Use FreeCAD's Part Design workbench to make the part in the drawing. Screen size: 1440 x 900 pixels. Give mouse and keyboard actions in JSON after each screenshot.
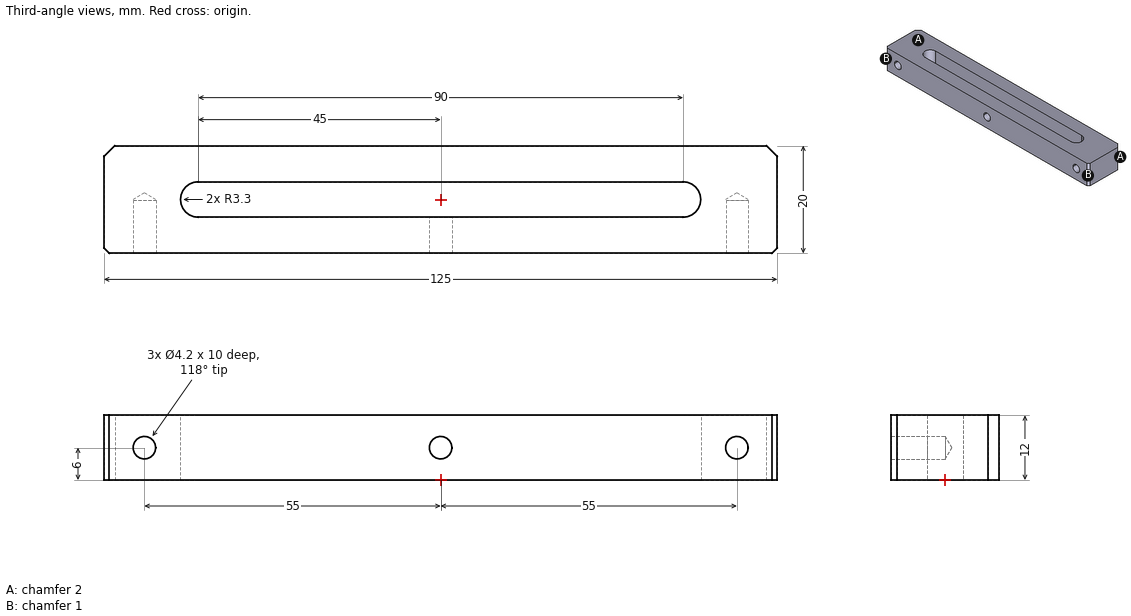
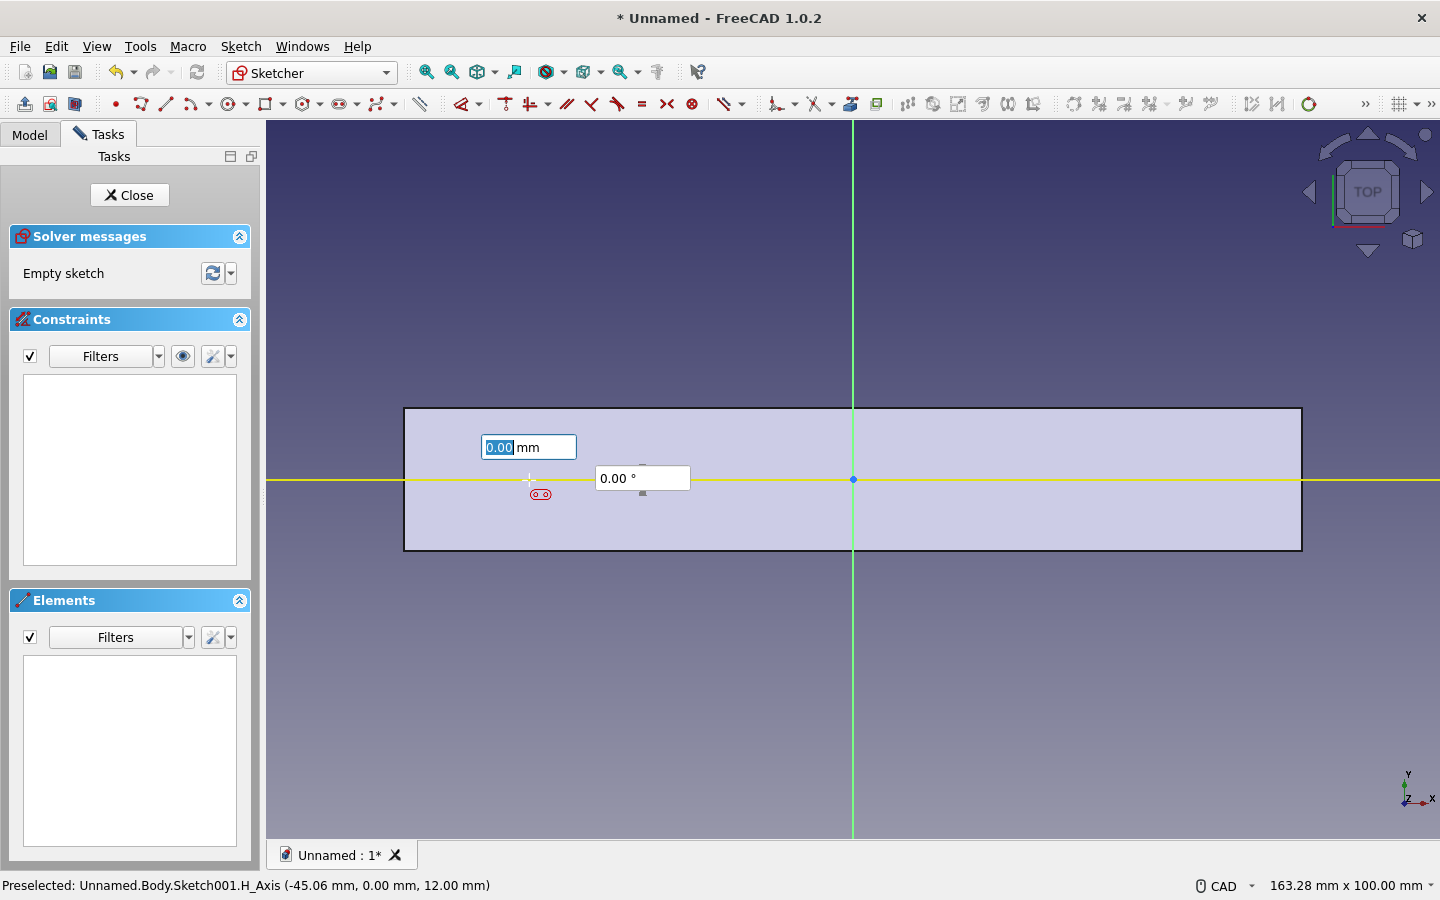
{"action": "left_click", "coordinate": [1177, 470]}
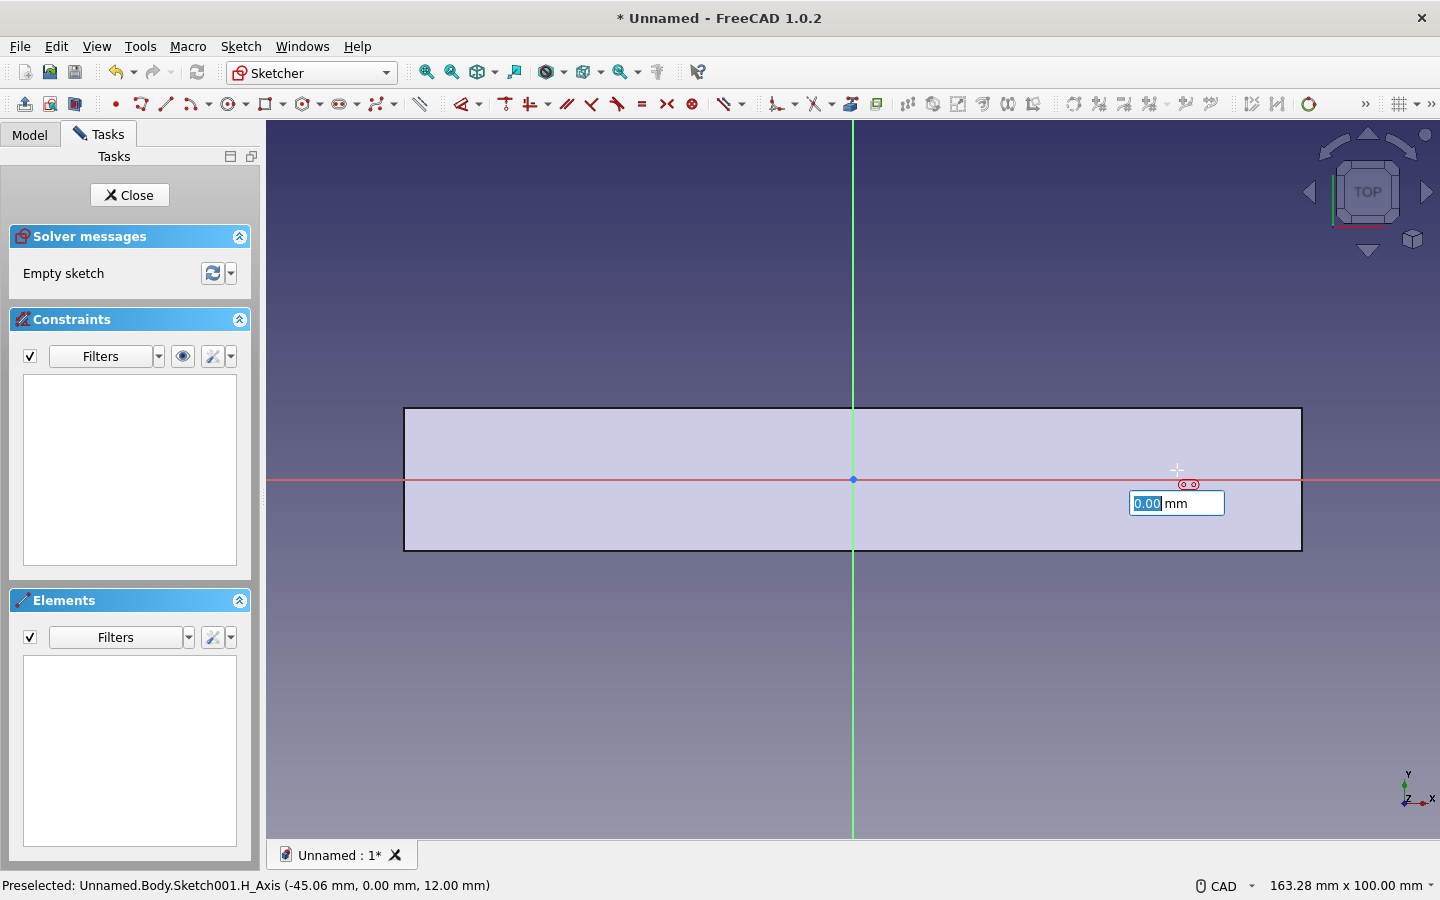
{"action": "left_click", "coordinate": [950, 456]}
{"action": "key", "text": "Escape"}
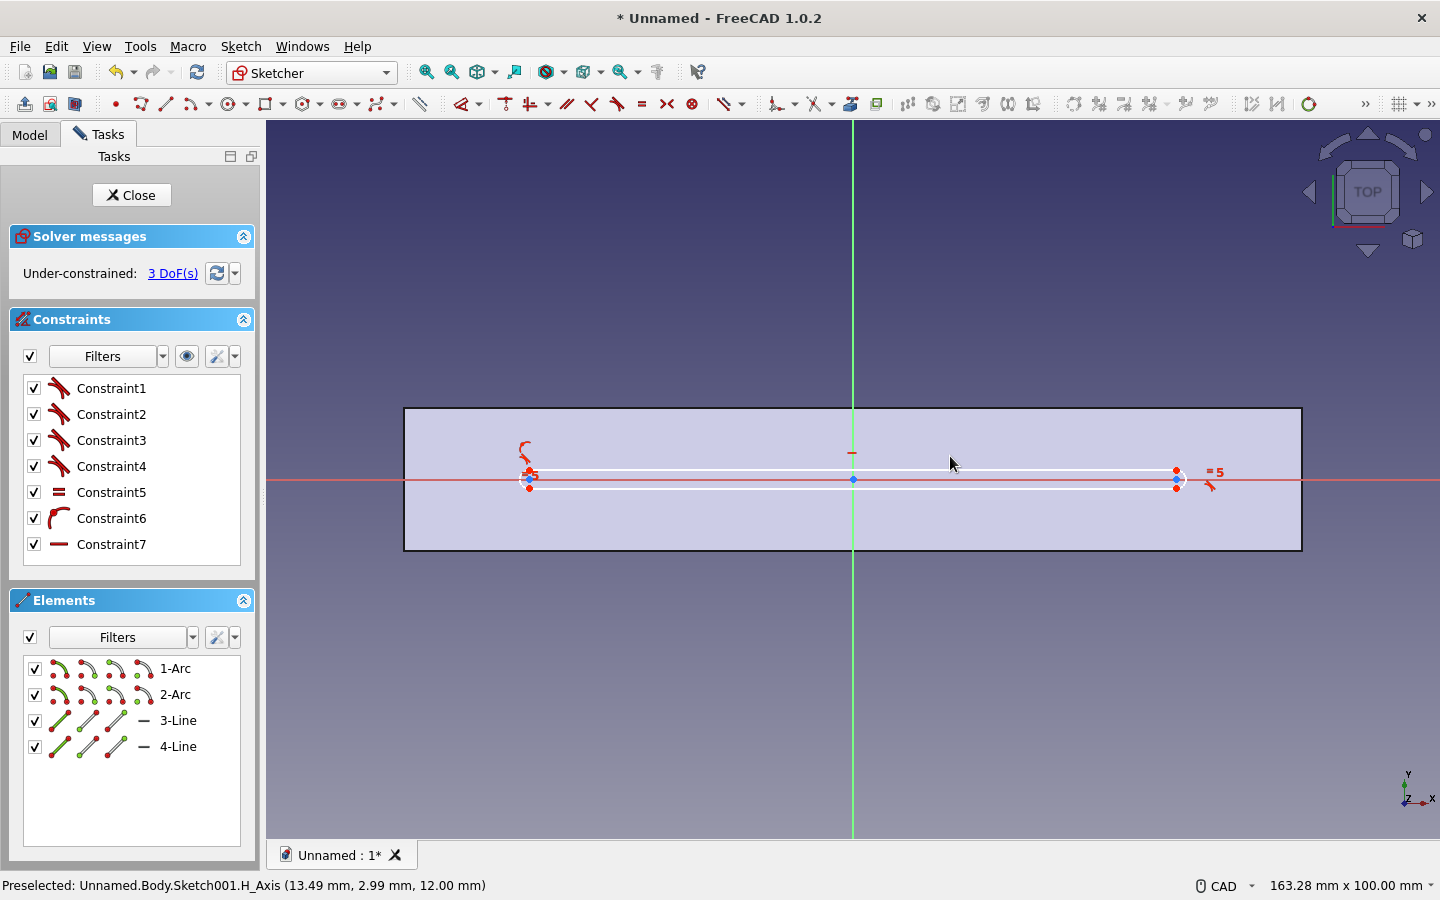
{"action": "key", "text": "d"}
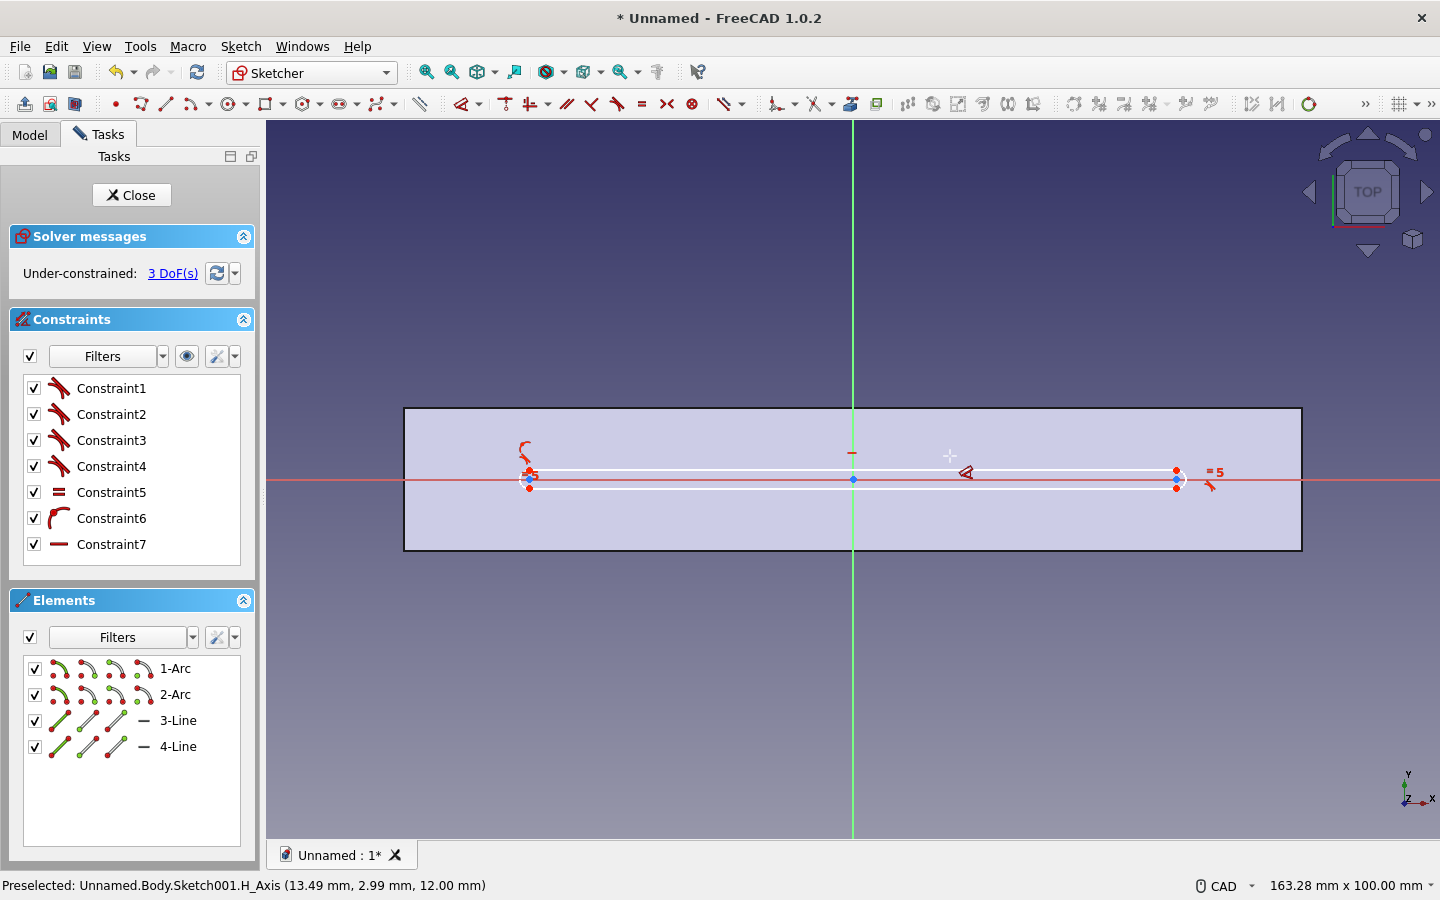
{"action": "scroll", "coordinate": [520, 479], "scroll_direction": "up", "scroll_amount": 3}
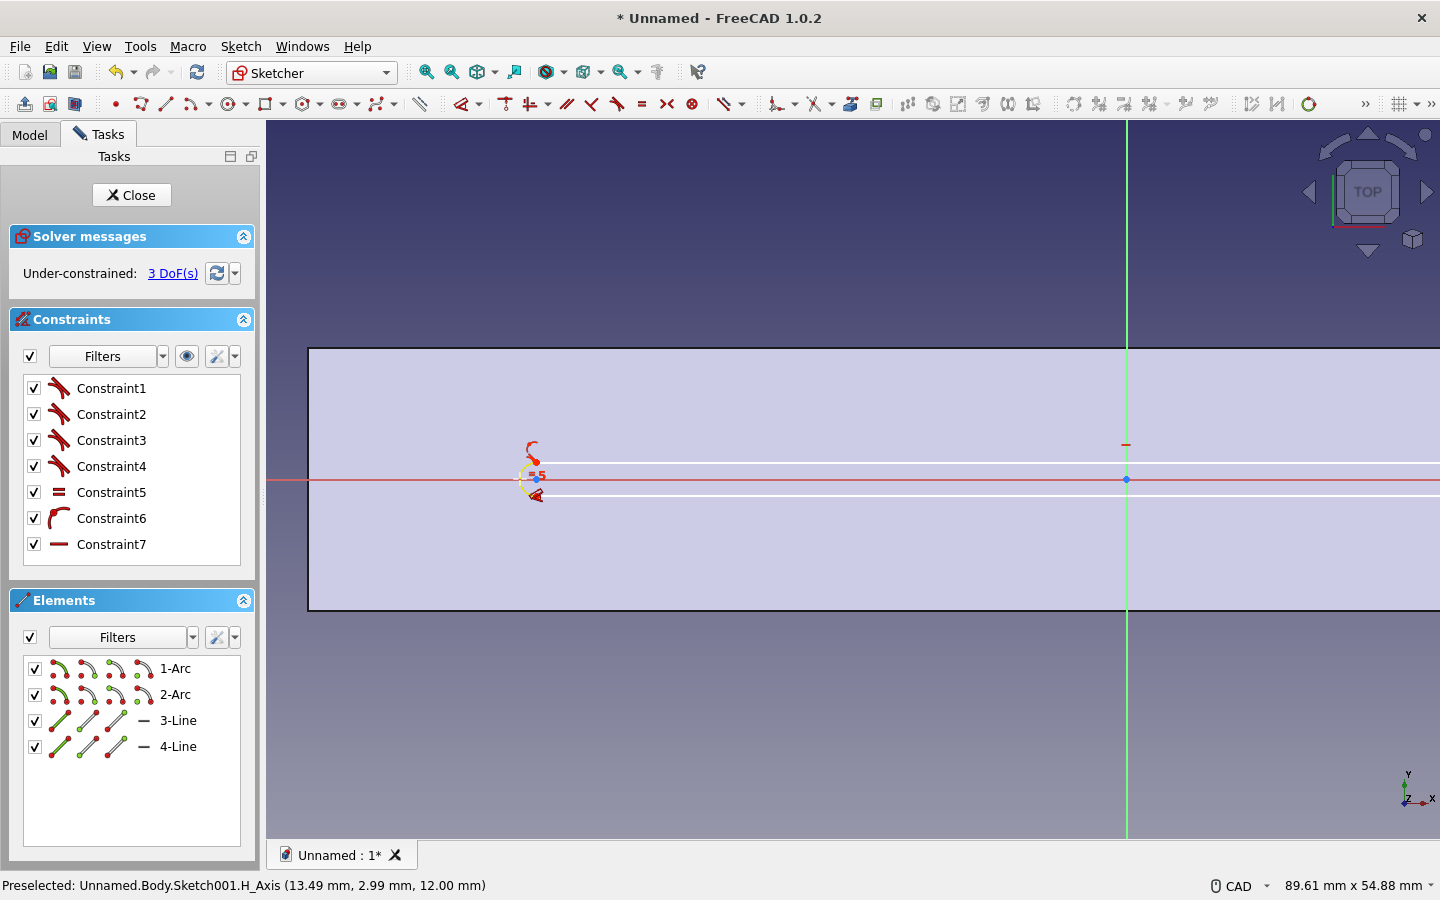
{"action": "left_click", "coordinate": [520, 479]}
{"action": "left_click", "coordinate": [495, 455]}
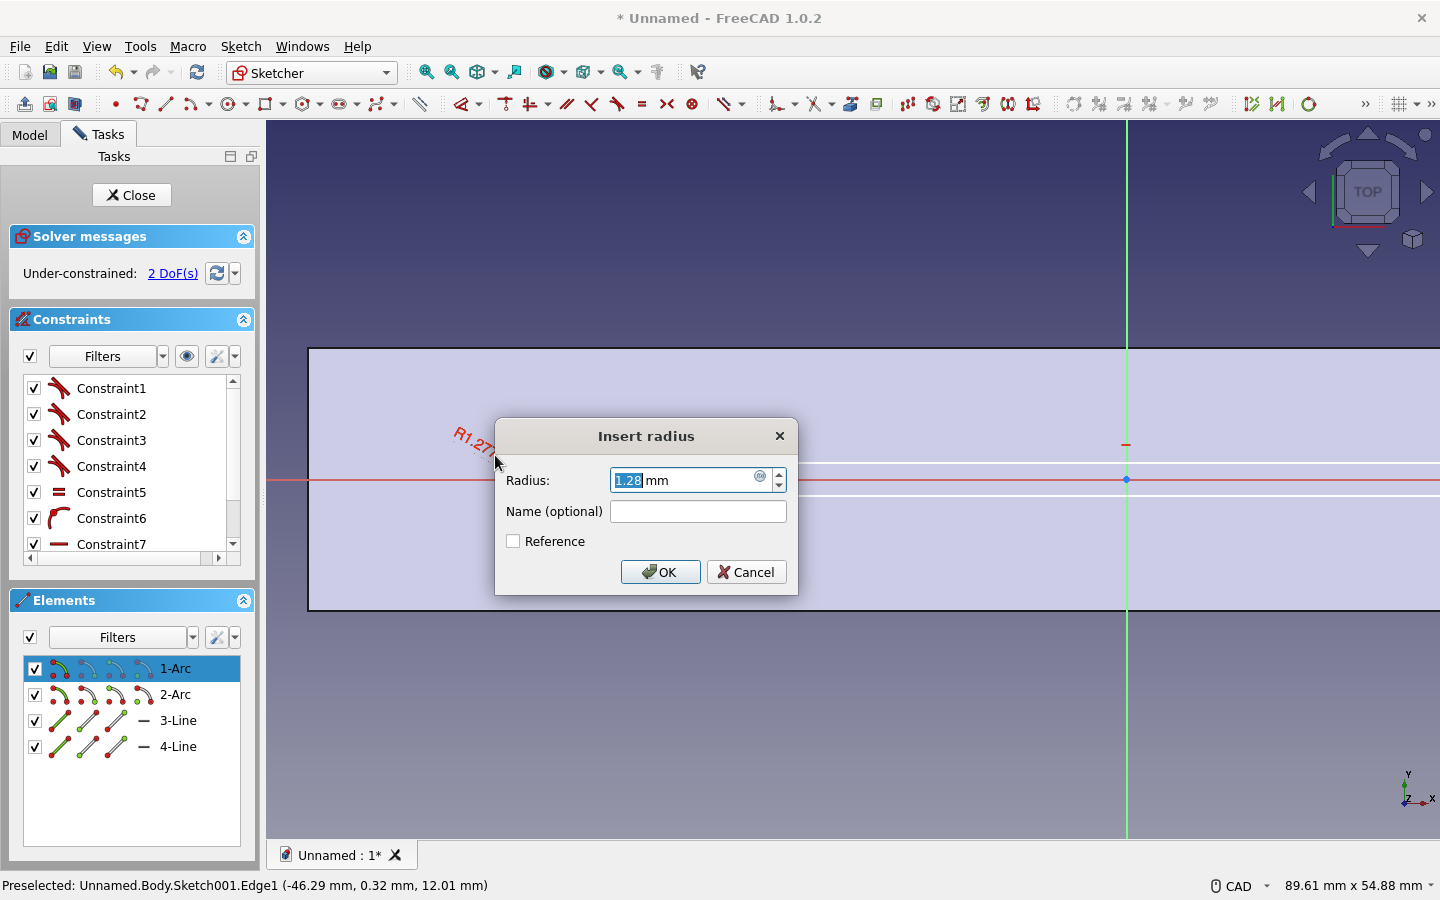
{"action": "type", "text": "3.3"}
{"action": "key", "text": "Return"}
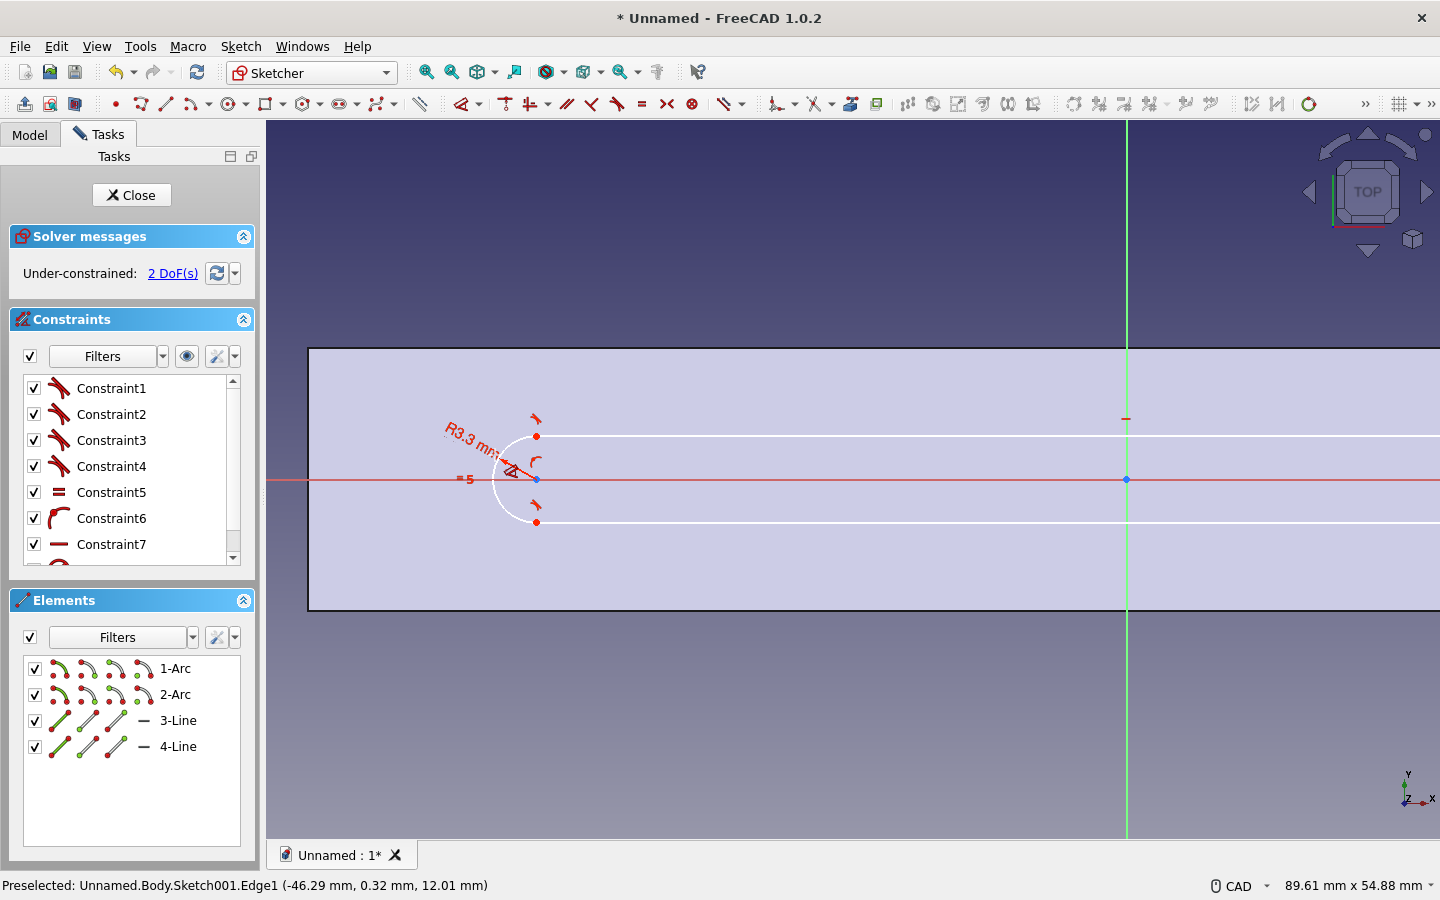
{"action": "left_click", "coordinate": [890, 436]}
{"action": "left_click", "coordinate": [906, 402]}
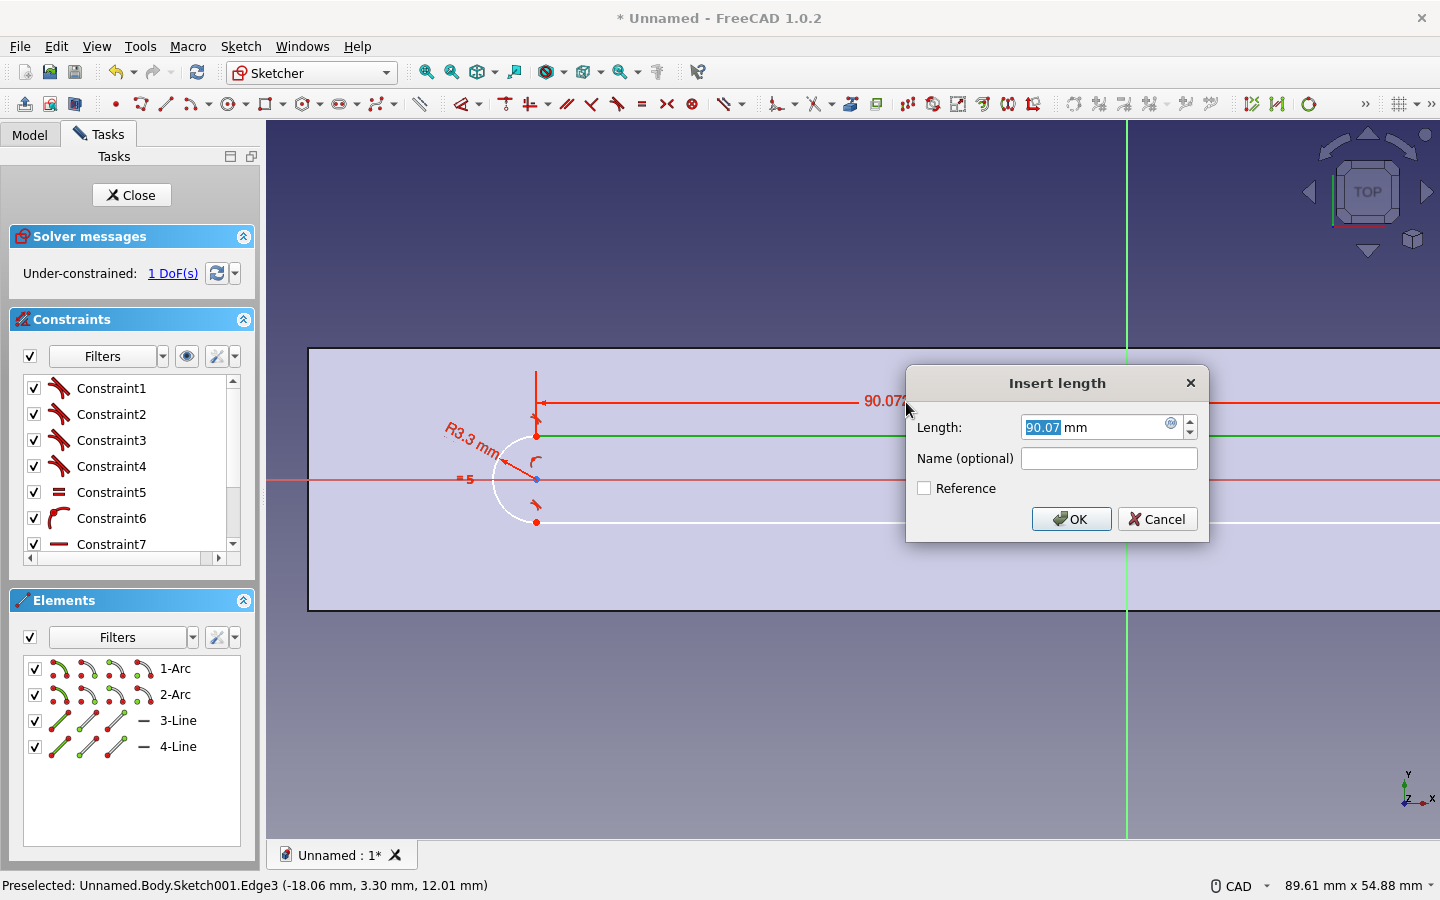
{"action": "type", "text": "90"}
{"action": "key", "text": "Return"}